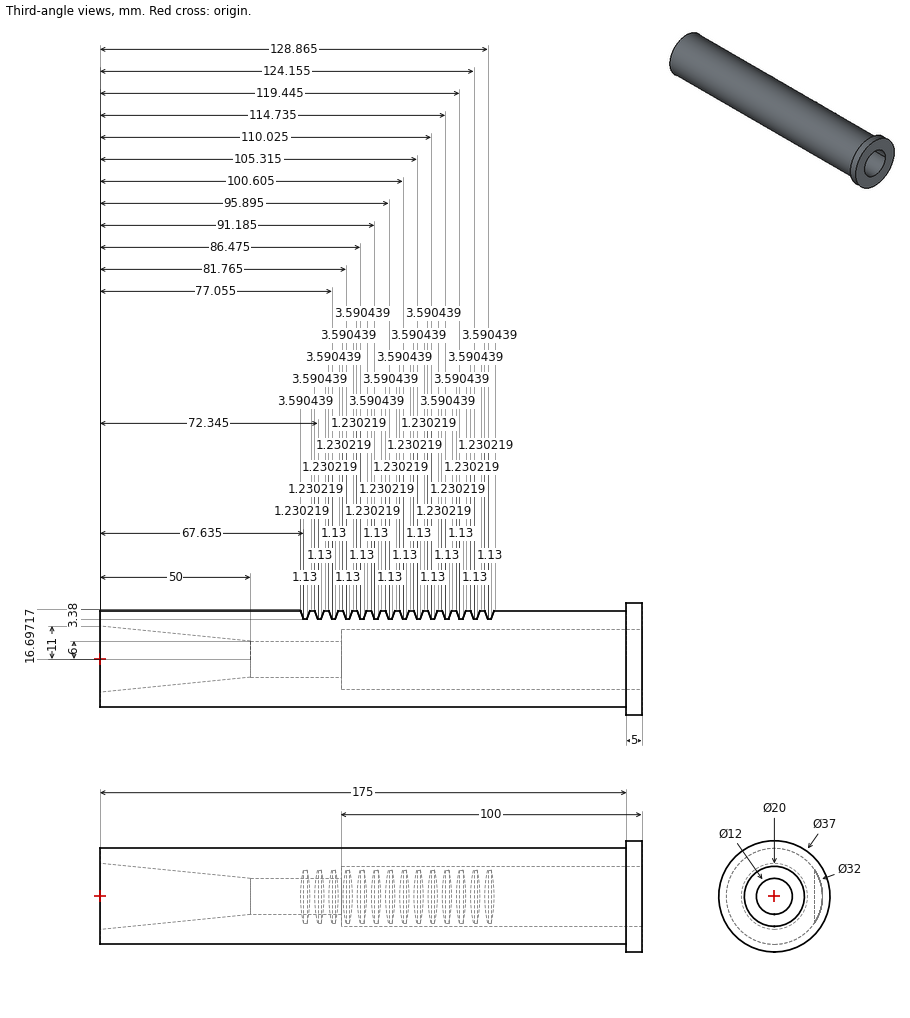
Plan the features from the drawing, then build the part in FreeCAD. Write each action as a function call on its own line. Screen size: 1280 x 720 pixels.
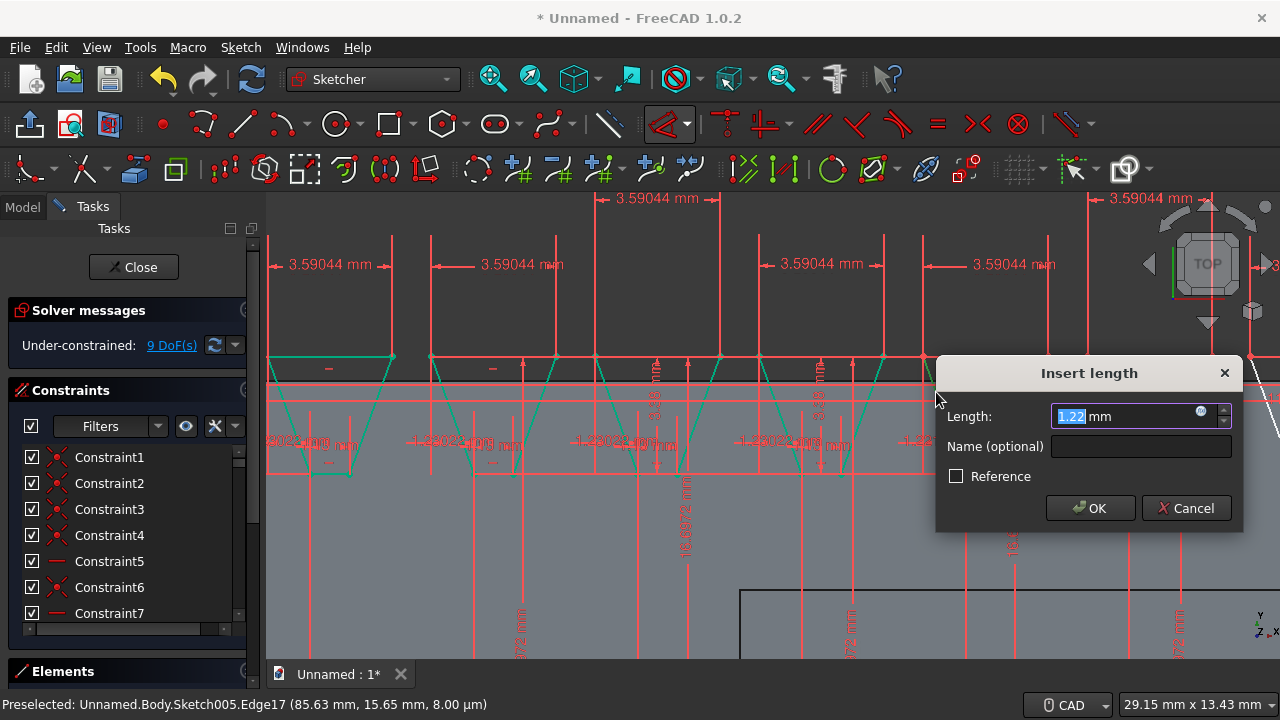
text(1.230219)
key(Return)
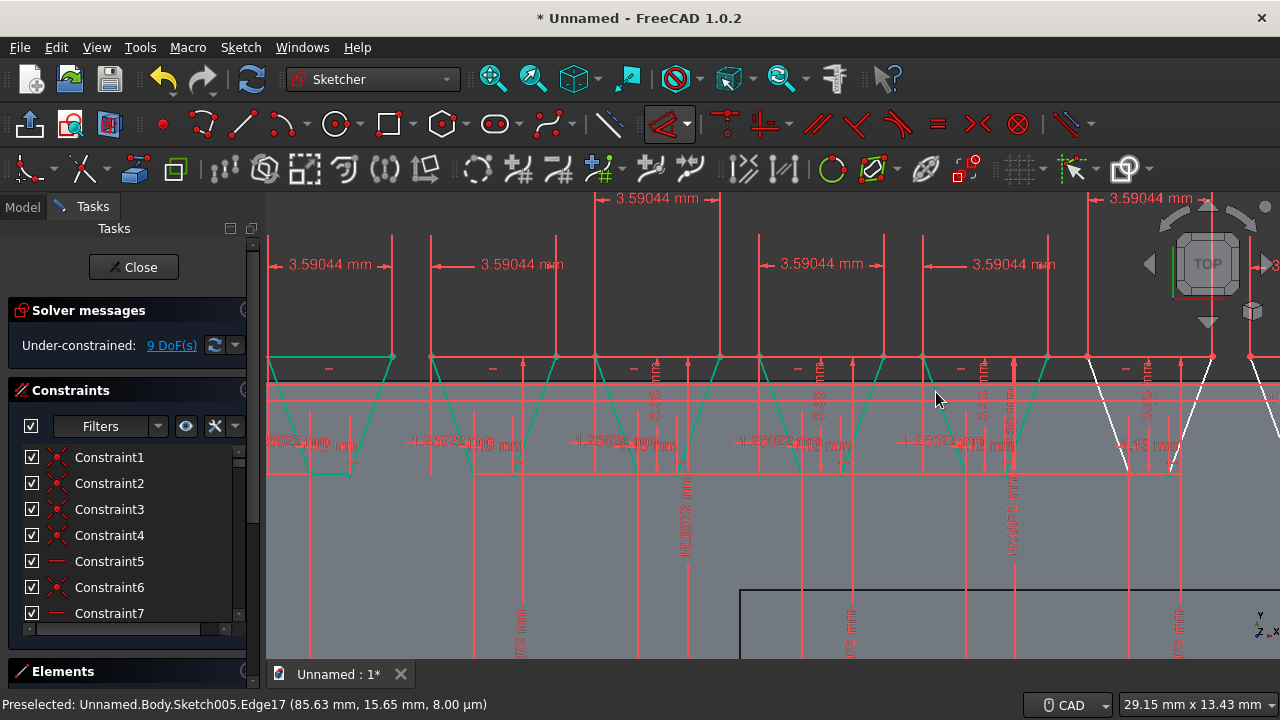
click(1100, 392)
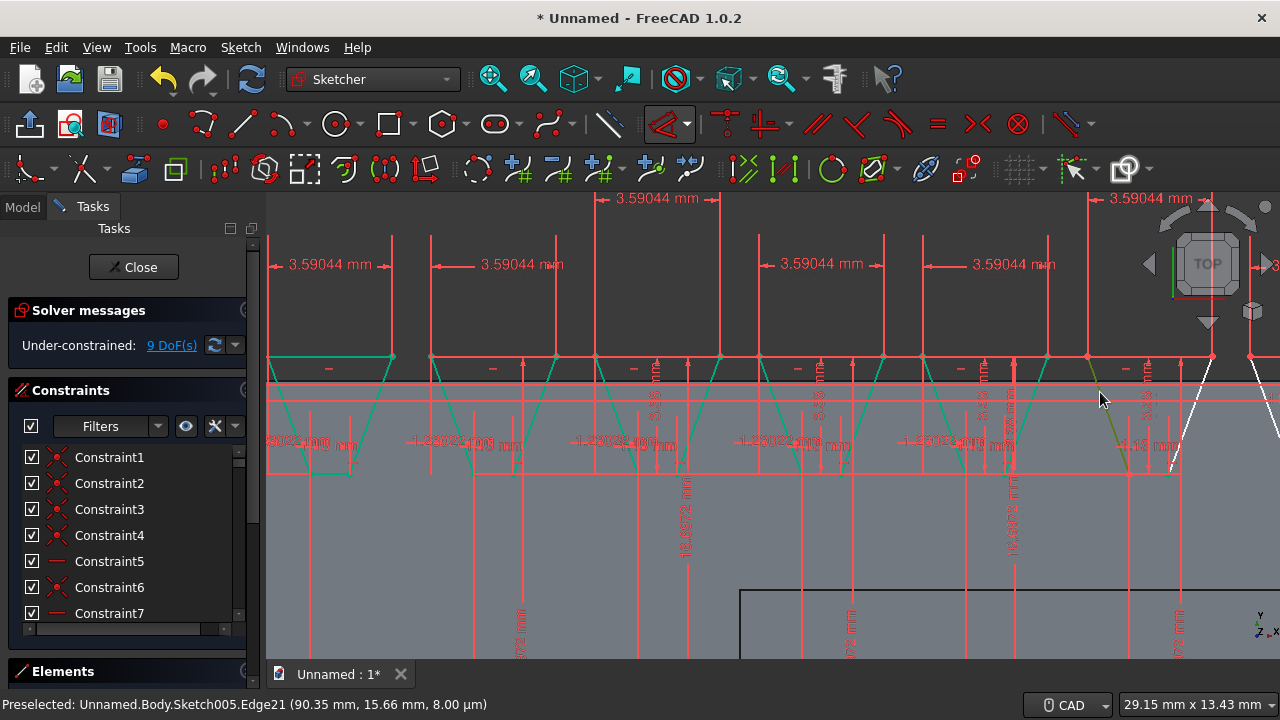
key(l)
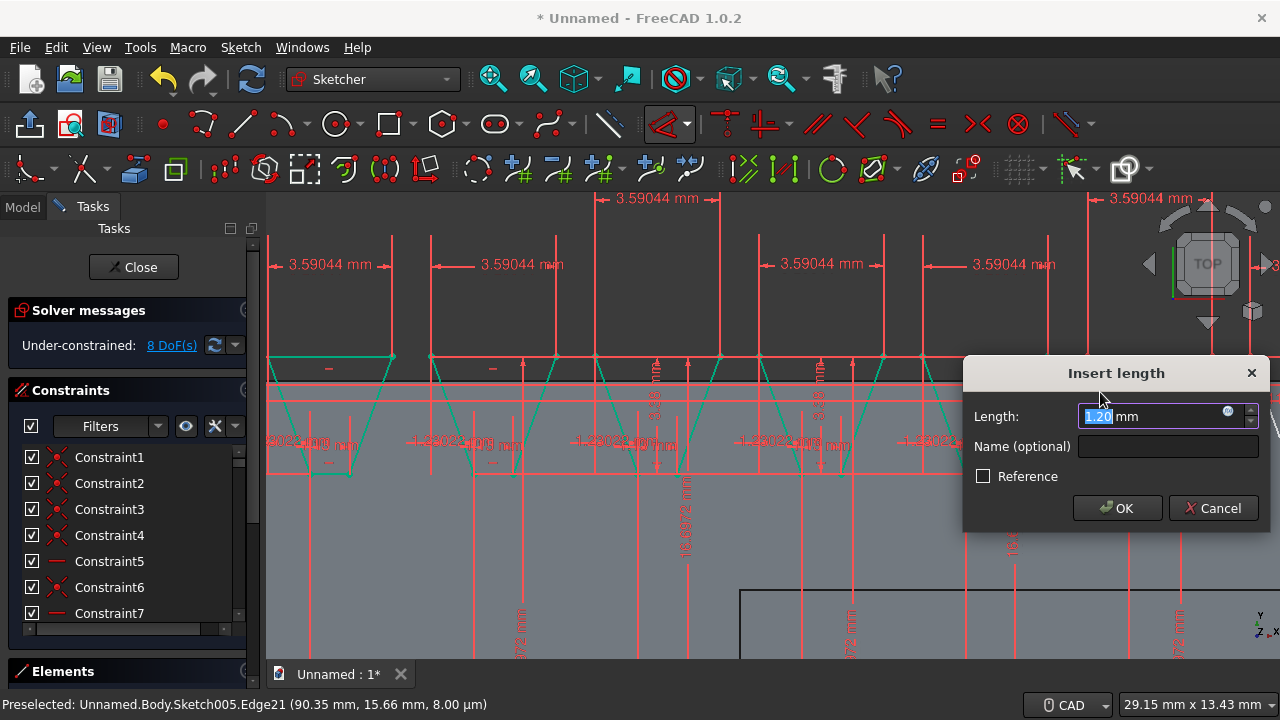
text(1.230219)
key(Return)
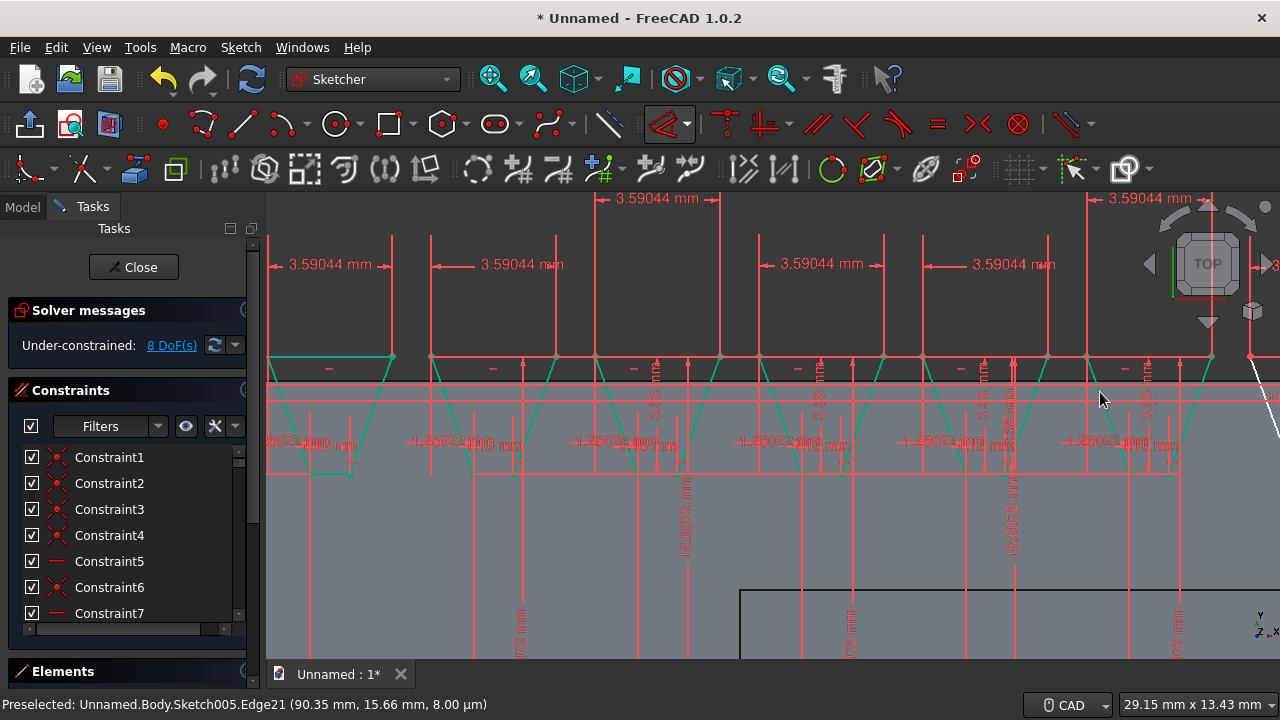
scroll(777, 391, down, 10)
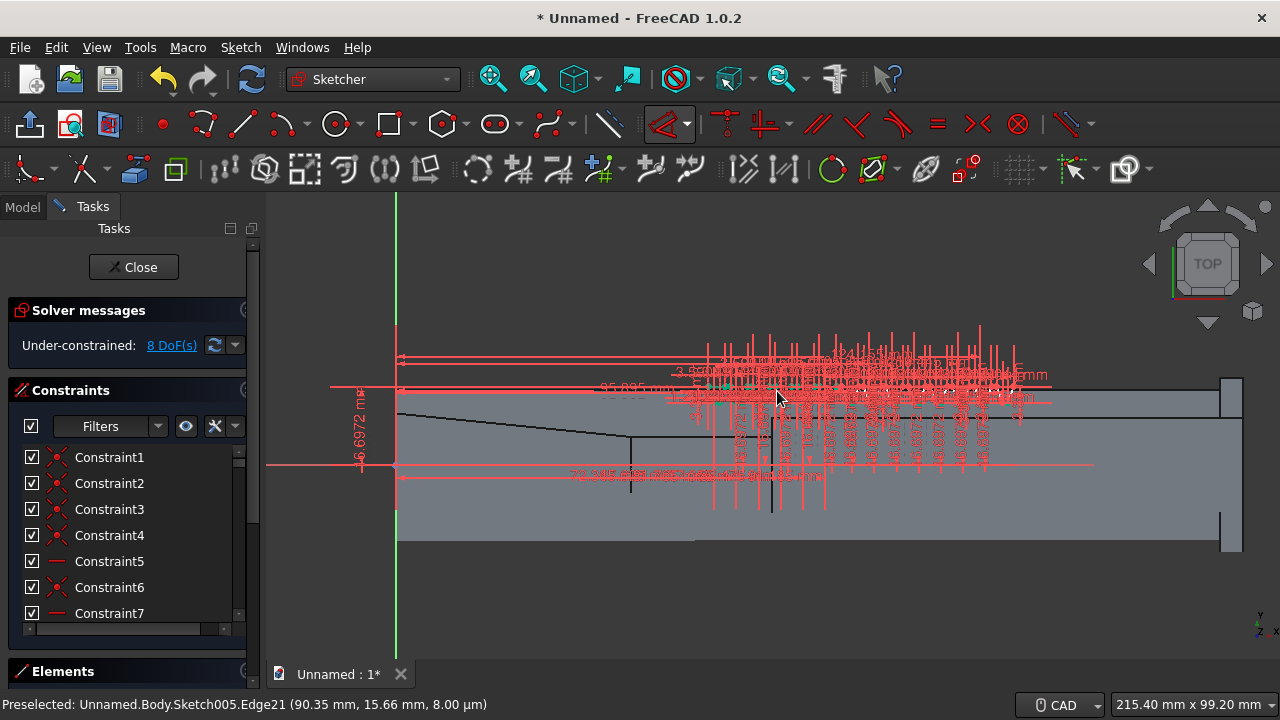
scroll(843, 391, up, 10)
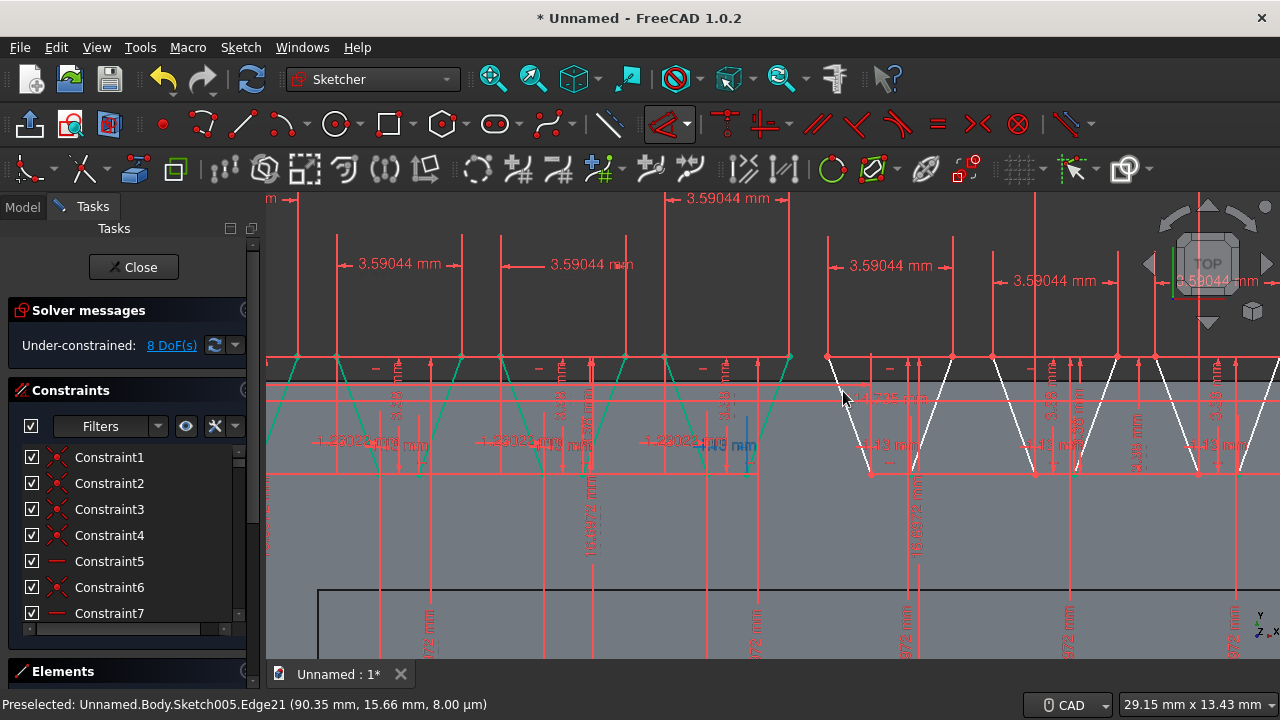
click(841, 392)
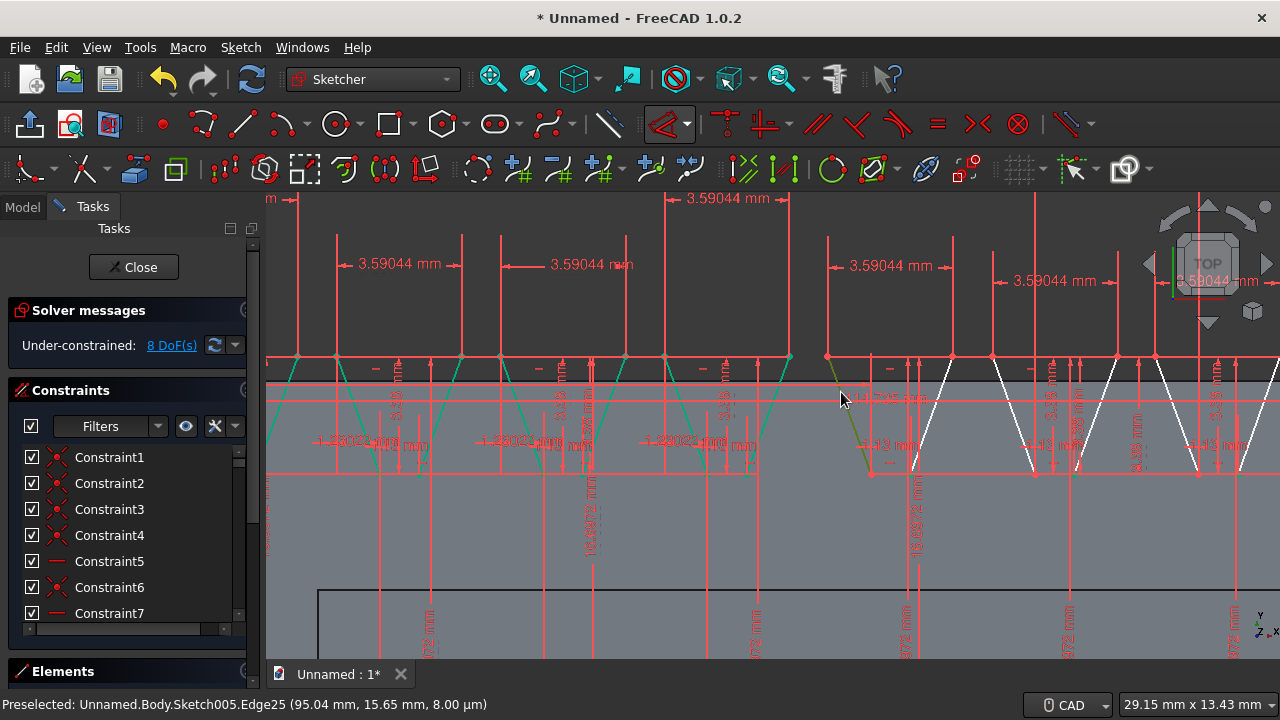
click(690, 124)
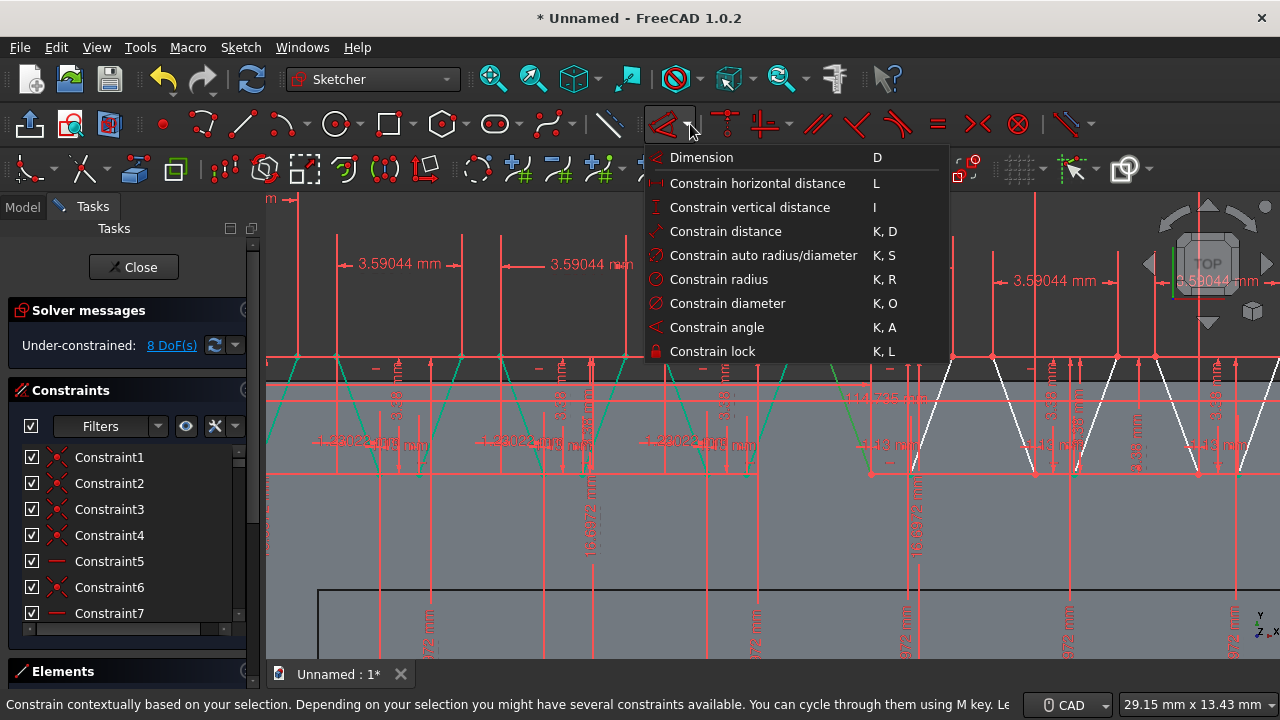
click(797, 183)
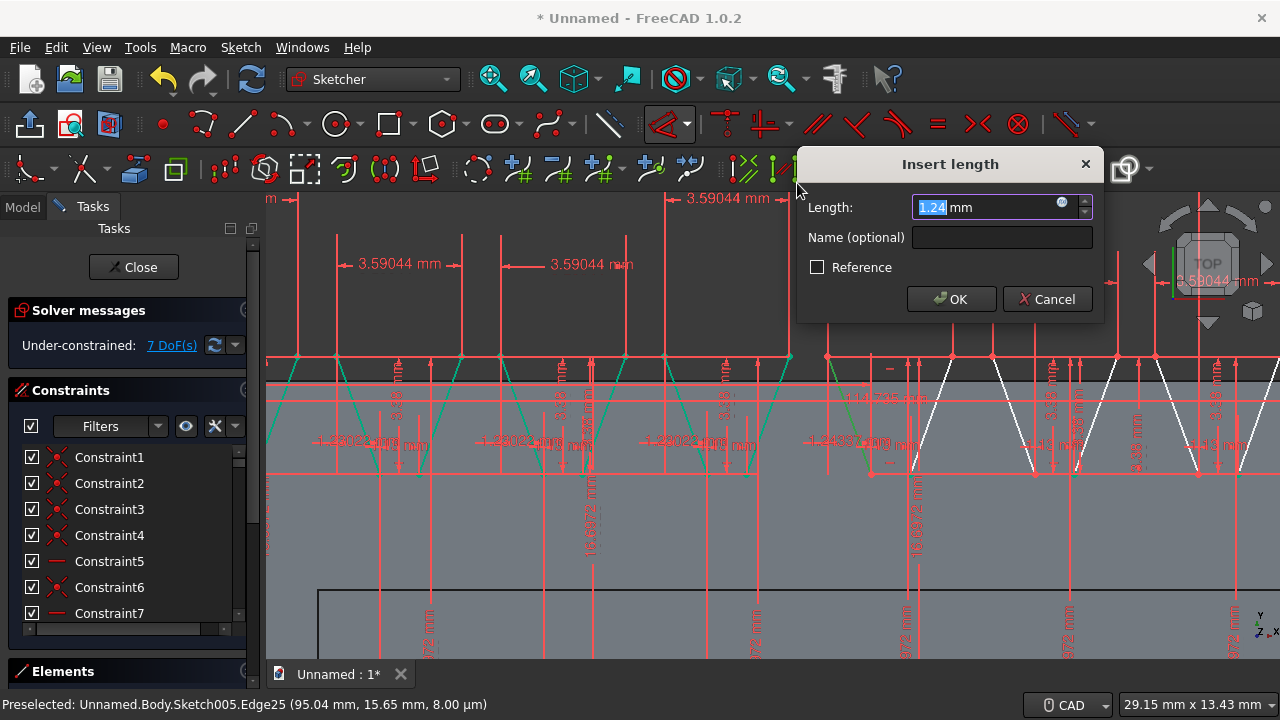
text(1.230219)
key(Return)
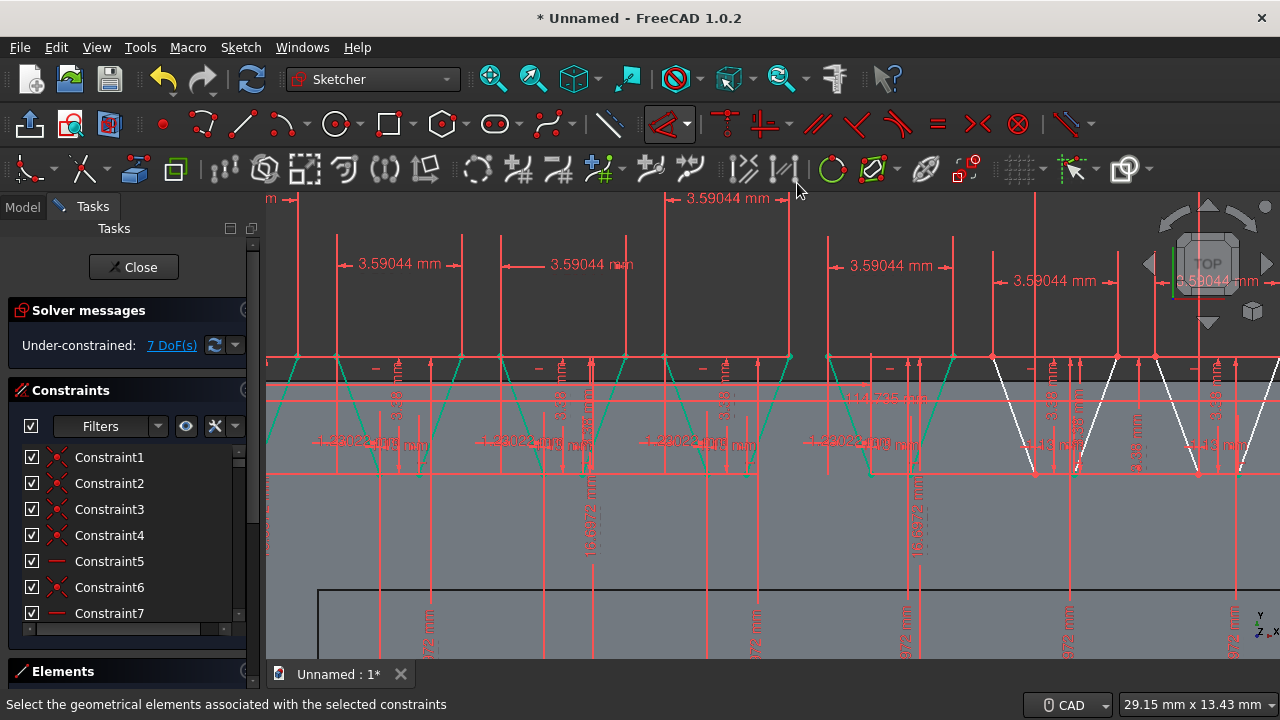
click(1005, 392)